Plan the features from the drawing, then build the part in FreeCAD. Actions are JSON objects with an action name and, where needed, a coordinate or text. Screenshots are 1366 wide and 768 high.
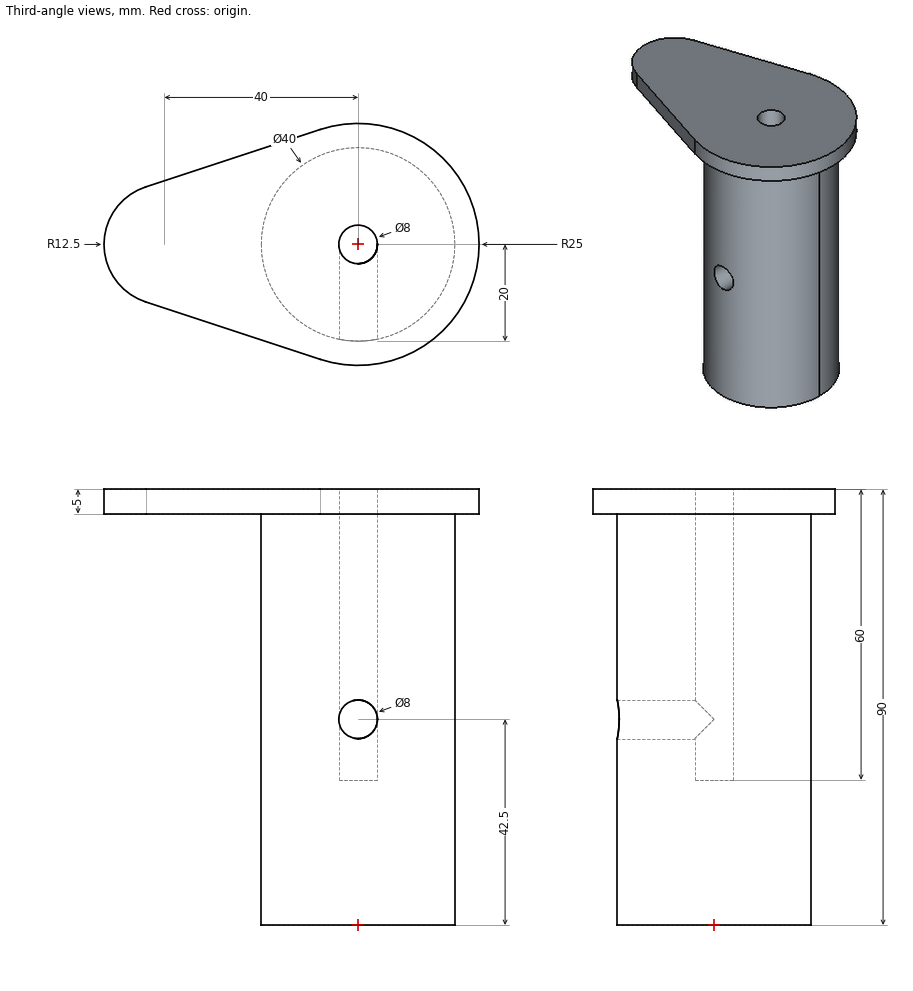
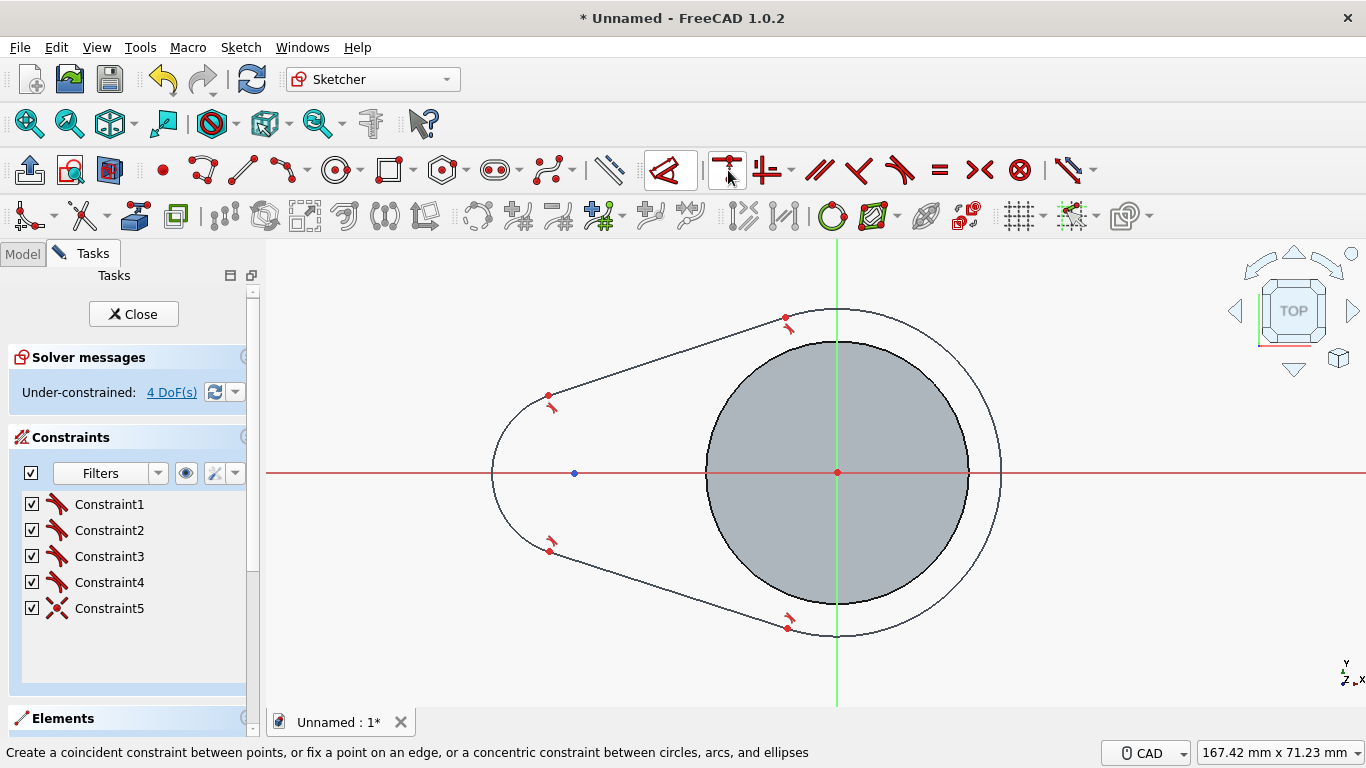
{"action": "left_click", "coordinate": [574, 474]}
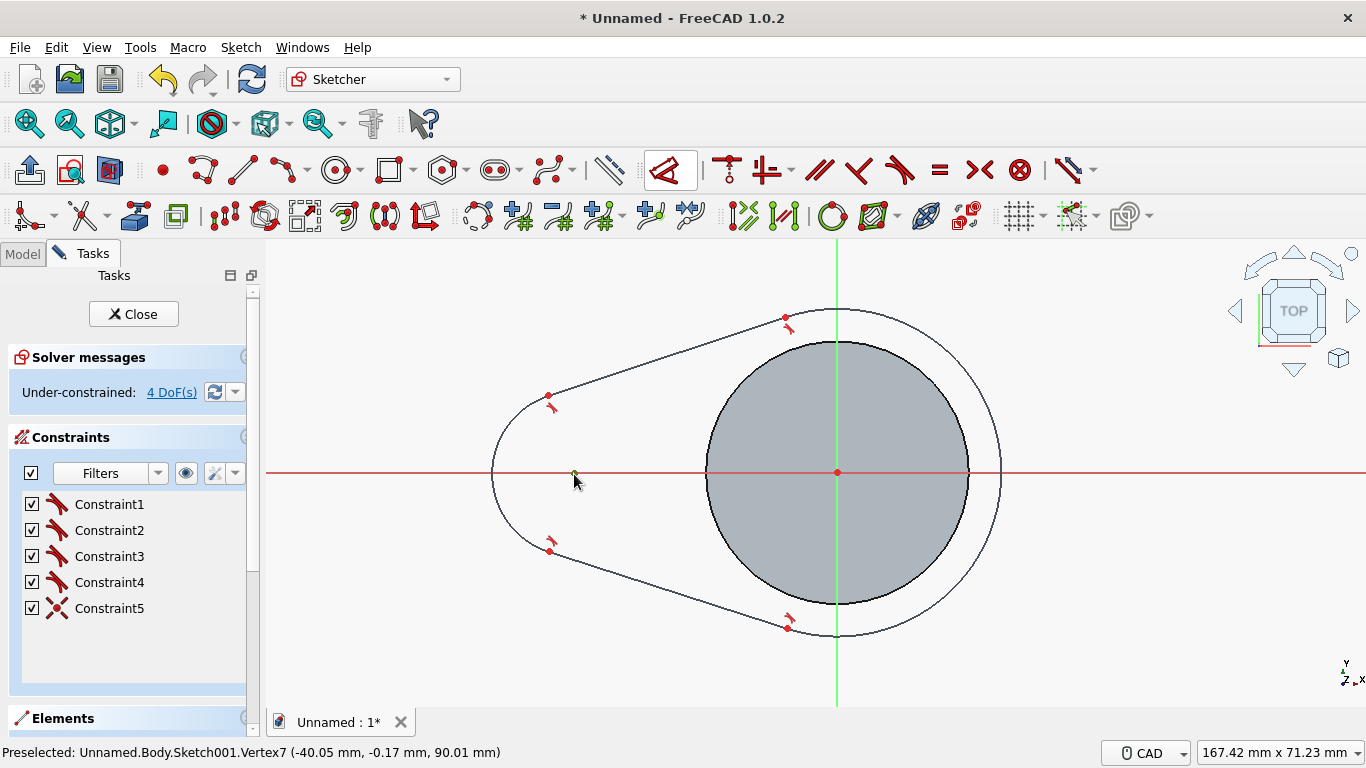
{"action": "left_click", "coordinate": [359, 473]}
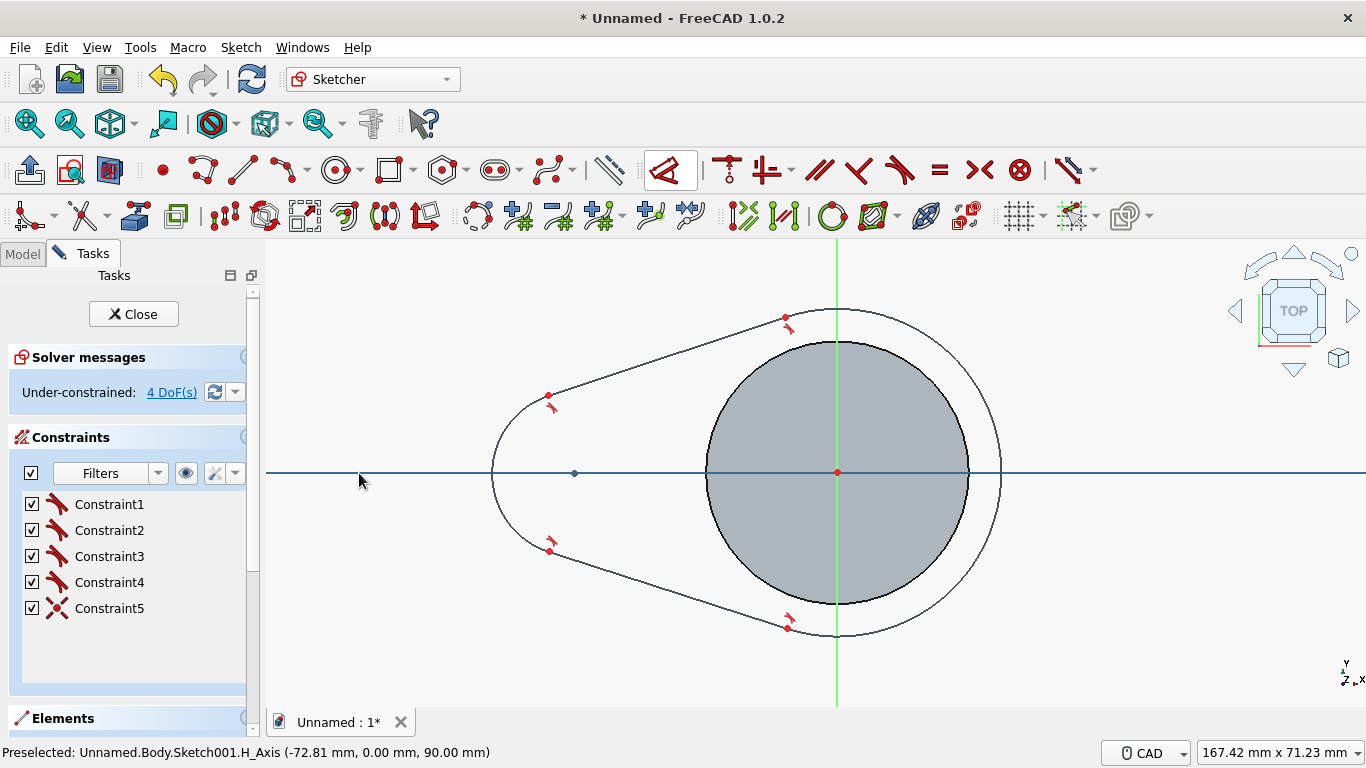
{"action": "key", "text": "c"}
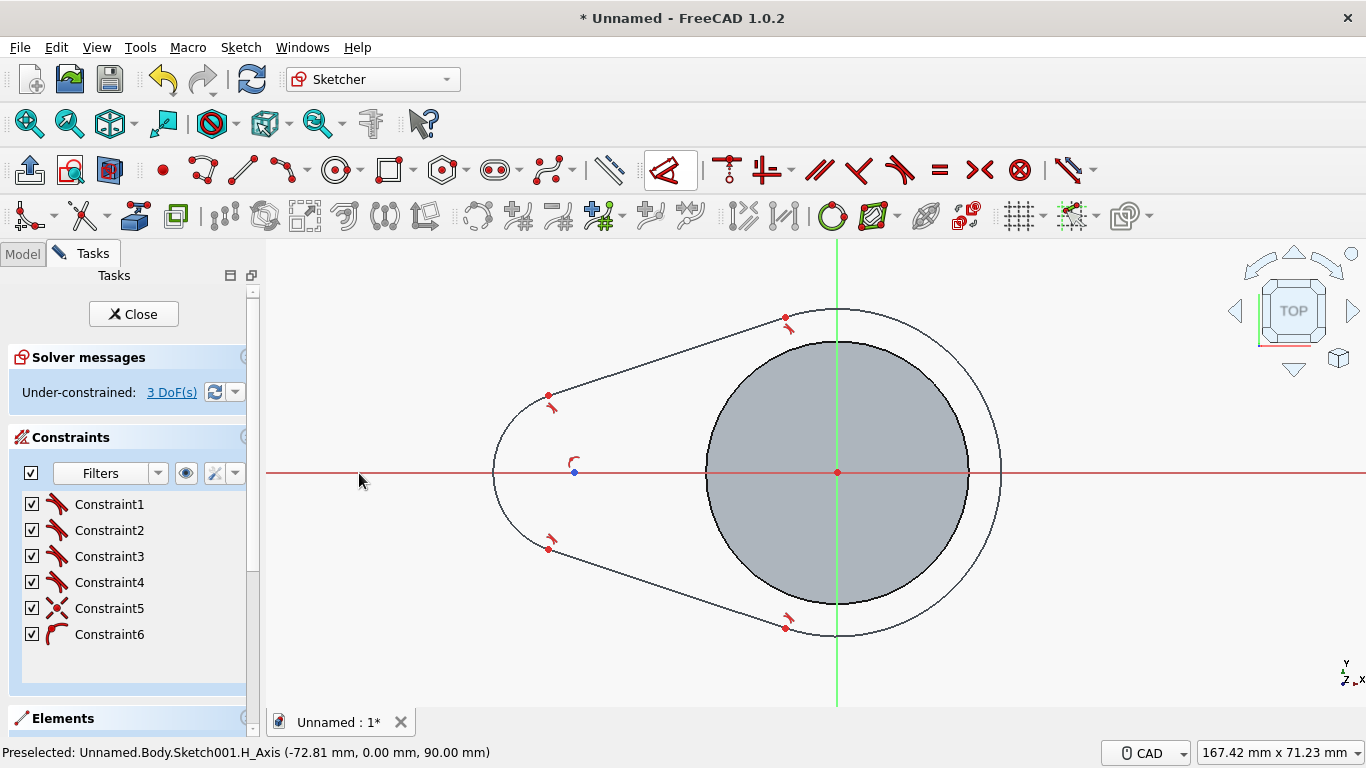
{"action": "left_click", "coordinate": [503, 434]}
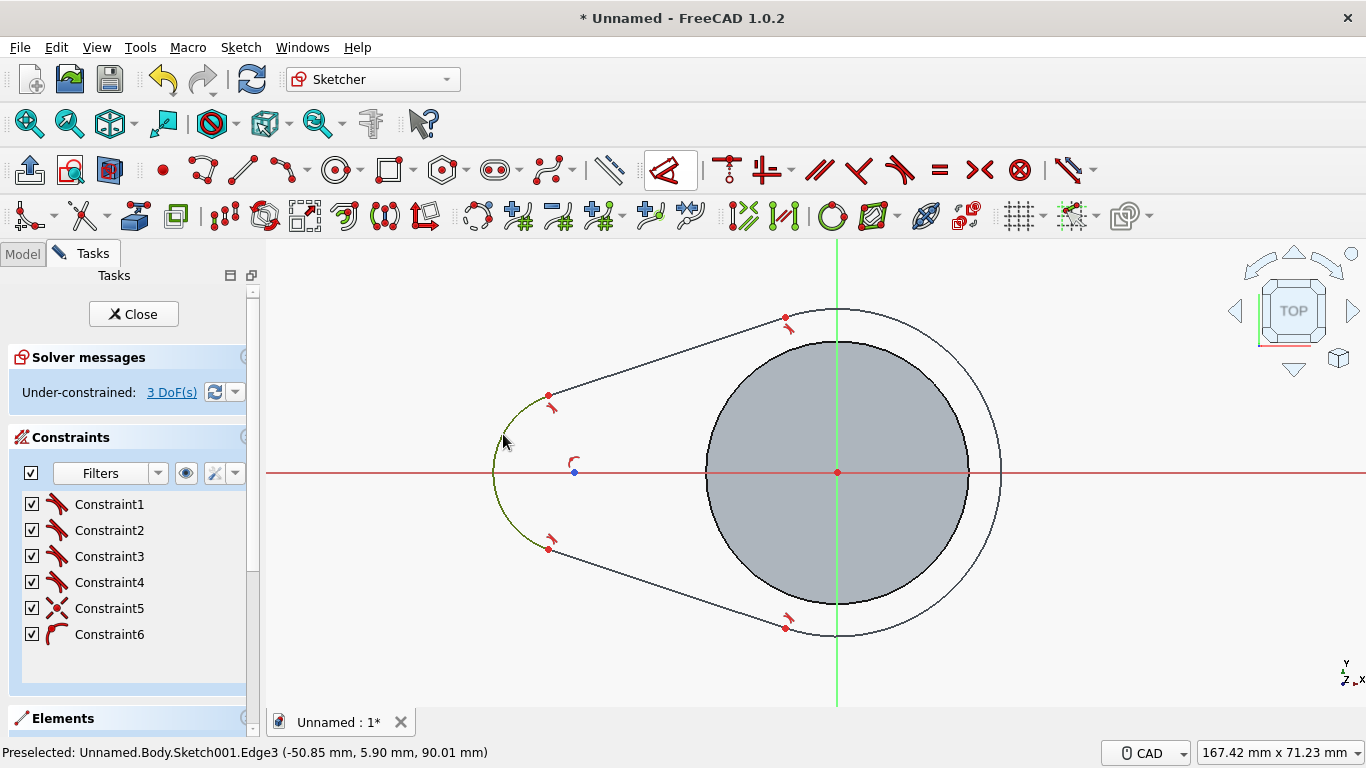
{"action": "key", "text": "k r"}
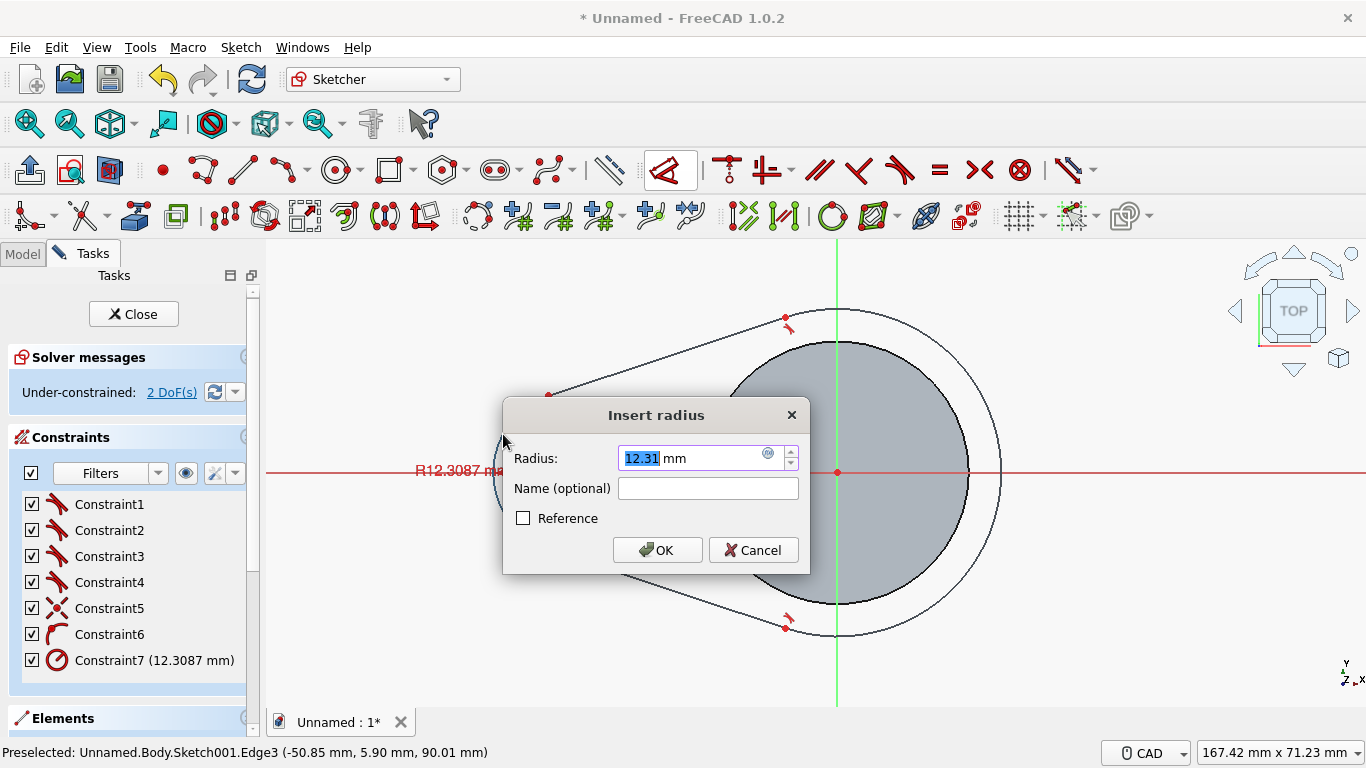
{"action": "type", "text": "12.5"}
{"action": "key", "text": "Return"}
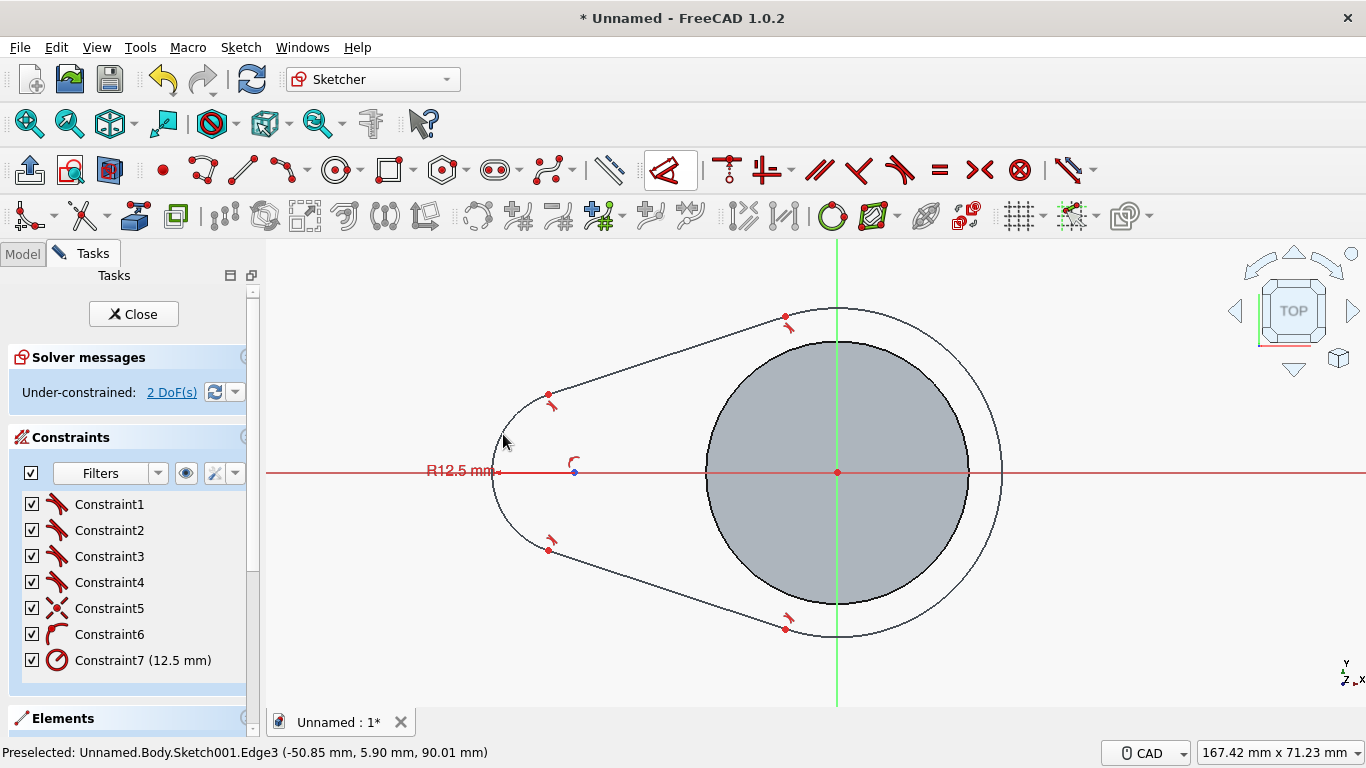
{"action": "left_click", "coordinate": [957, 586]}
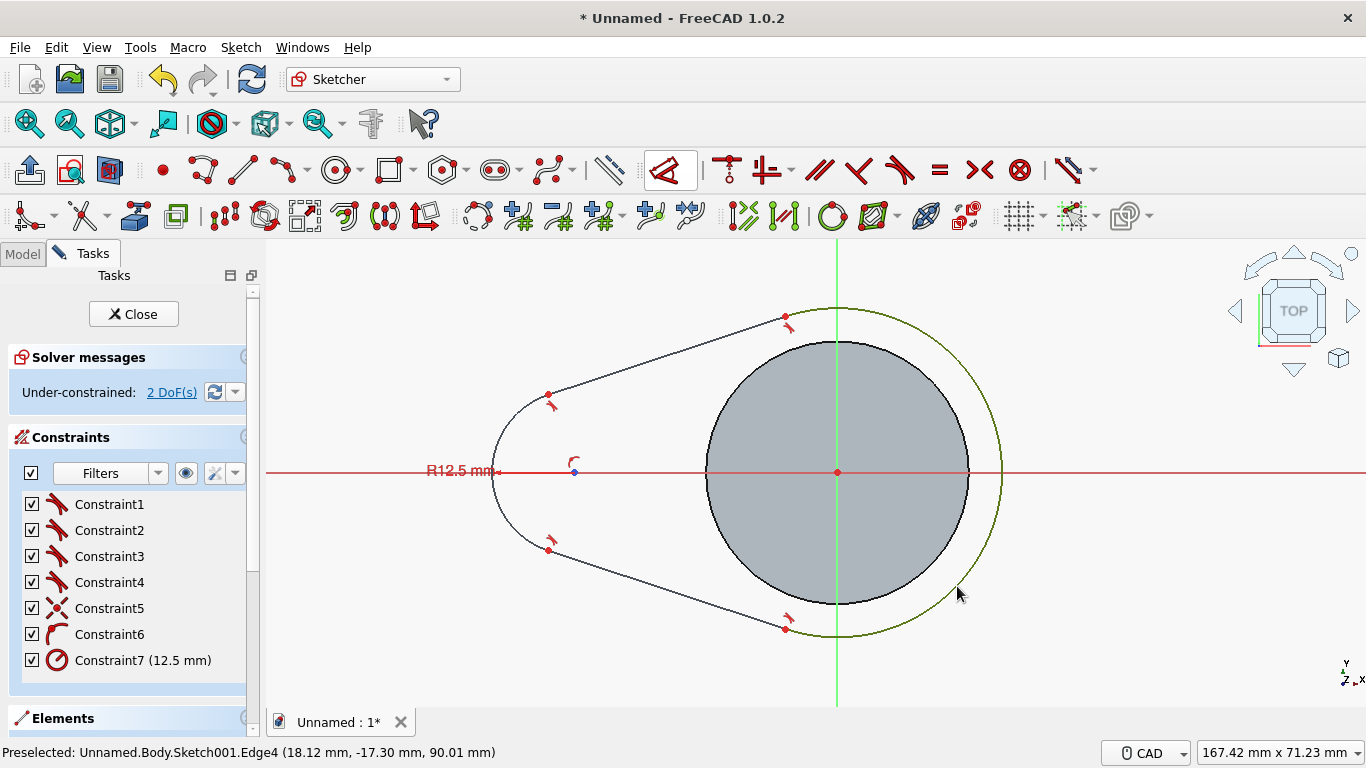
{"action": "key", "text": "k r"}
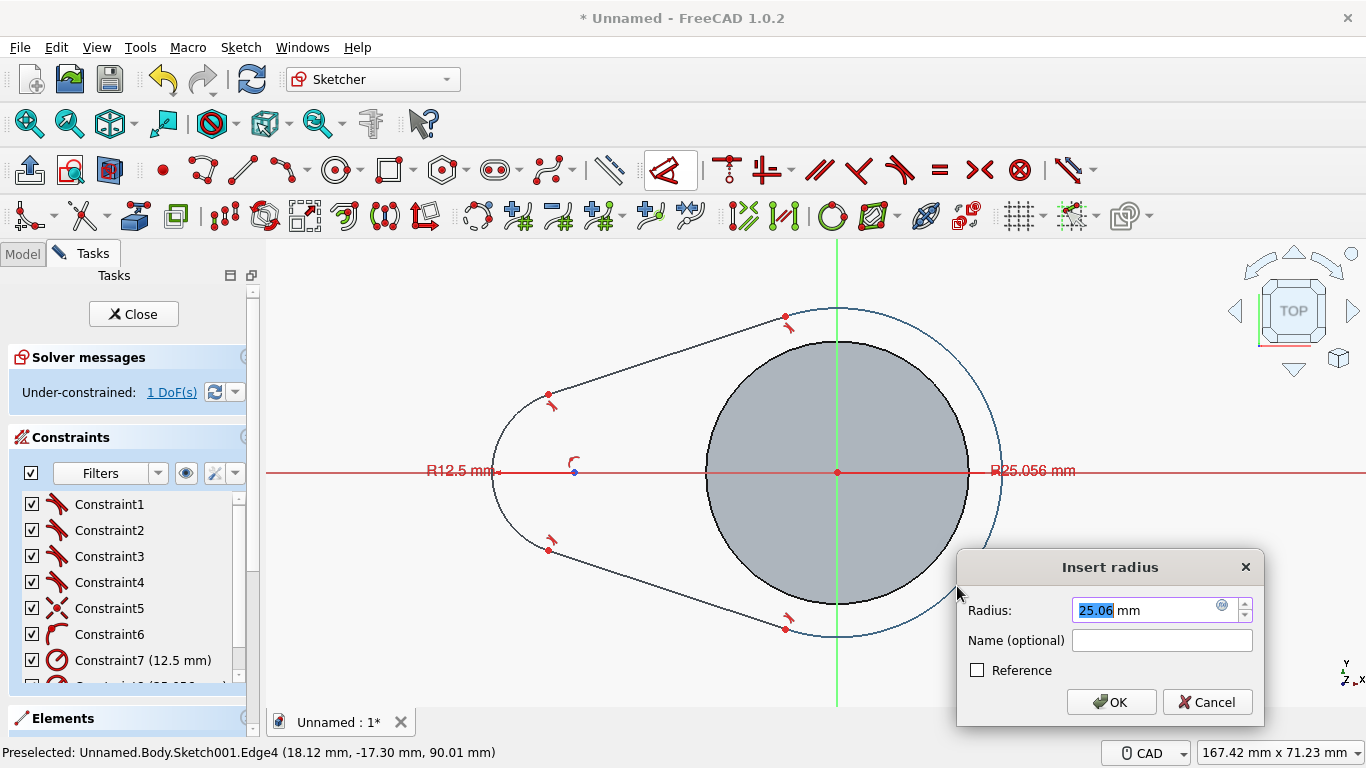
{"action": "type", "text": "25"}
{"action": "key", "text": "Return"}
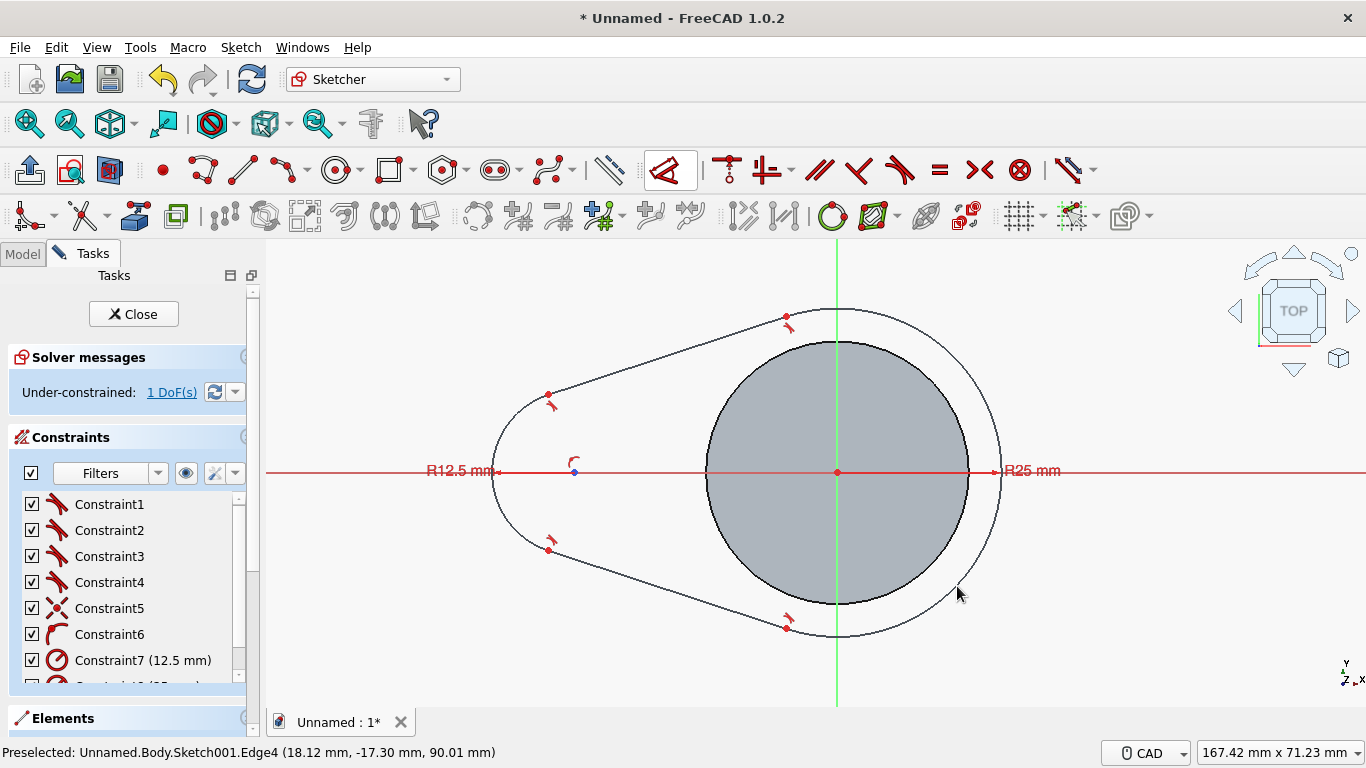
{"action": "left_click", "coordinate": [574, 473]}